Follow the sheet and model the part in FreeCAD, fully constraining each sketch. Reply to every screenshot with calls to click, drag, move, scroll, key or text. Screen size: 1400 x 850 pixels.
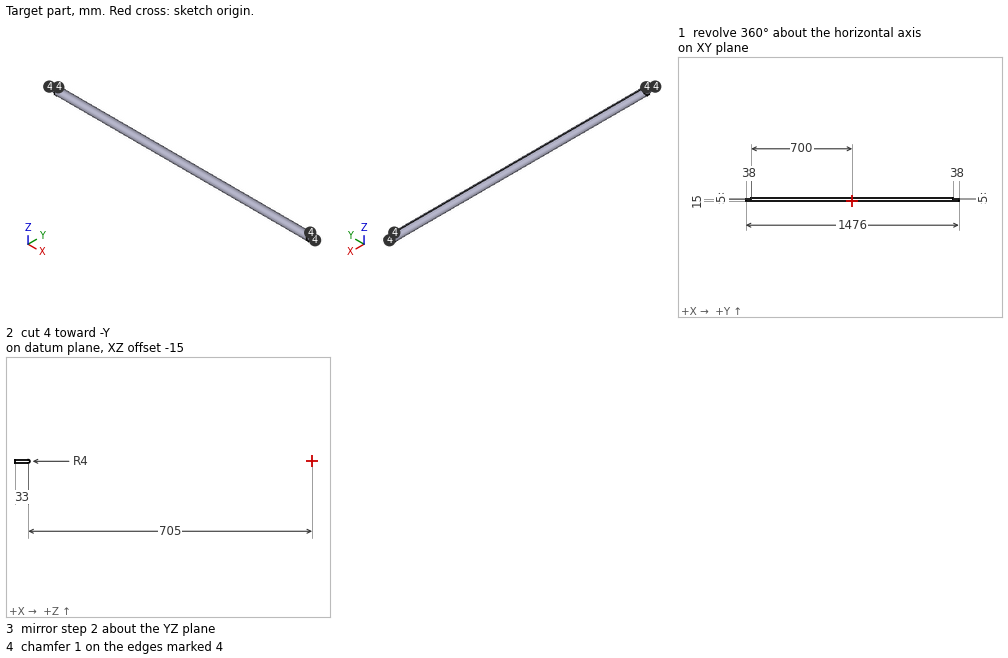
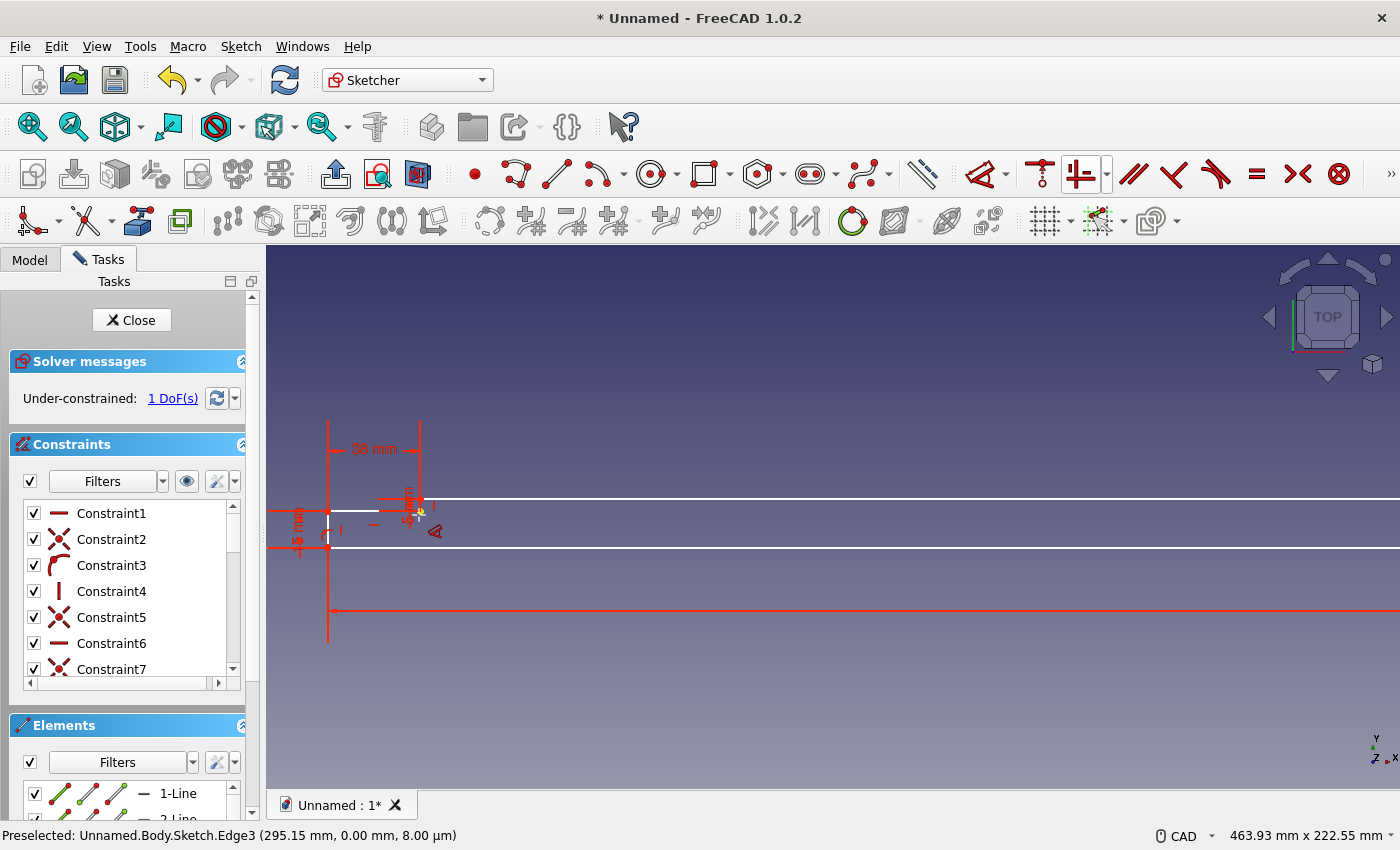
click(420, 511)
click(828, 582)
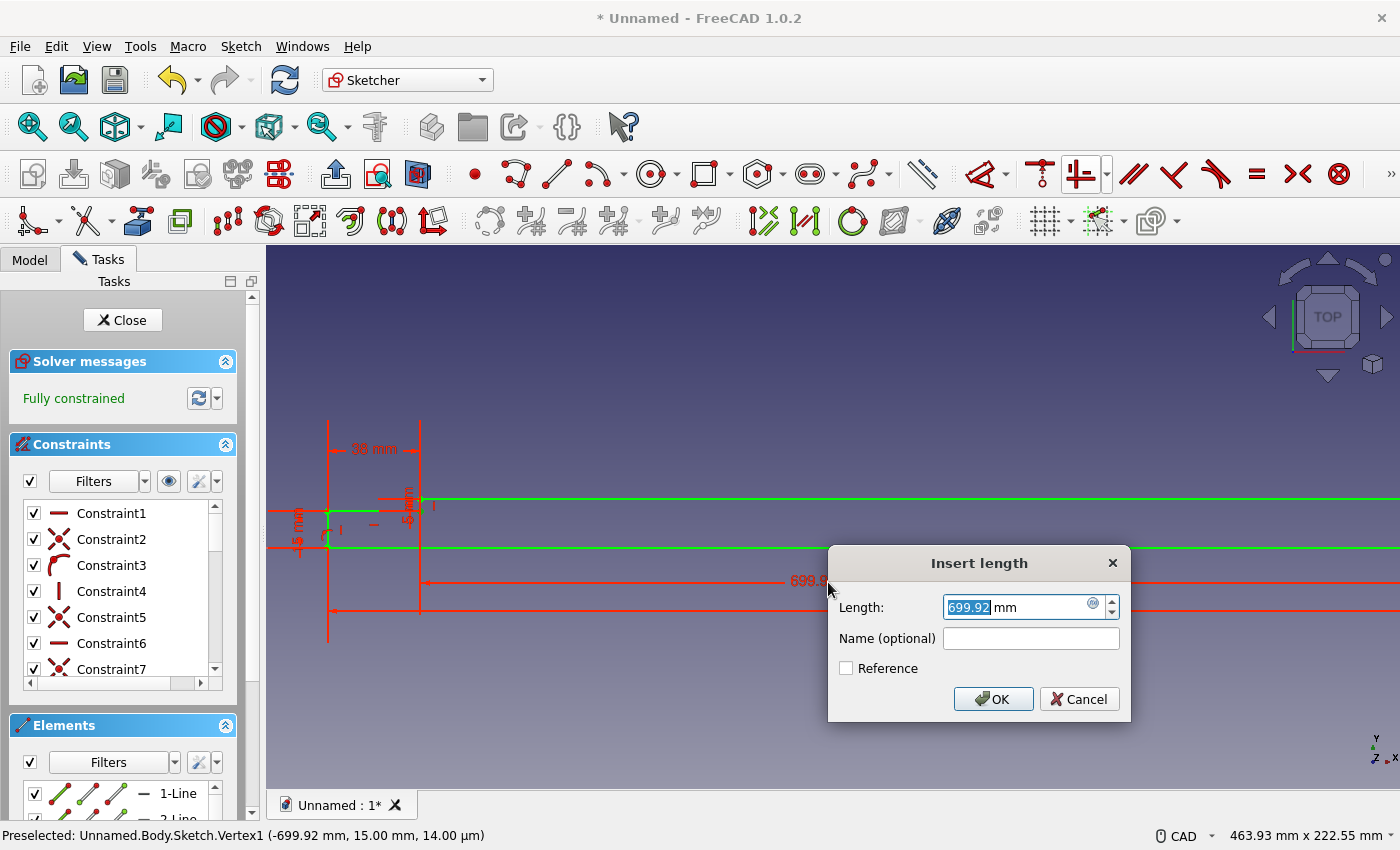
text(700)
key(Return)
key(Escape)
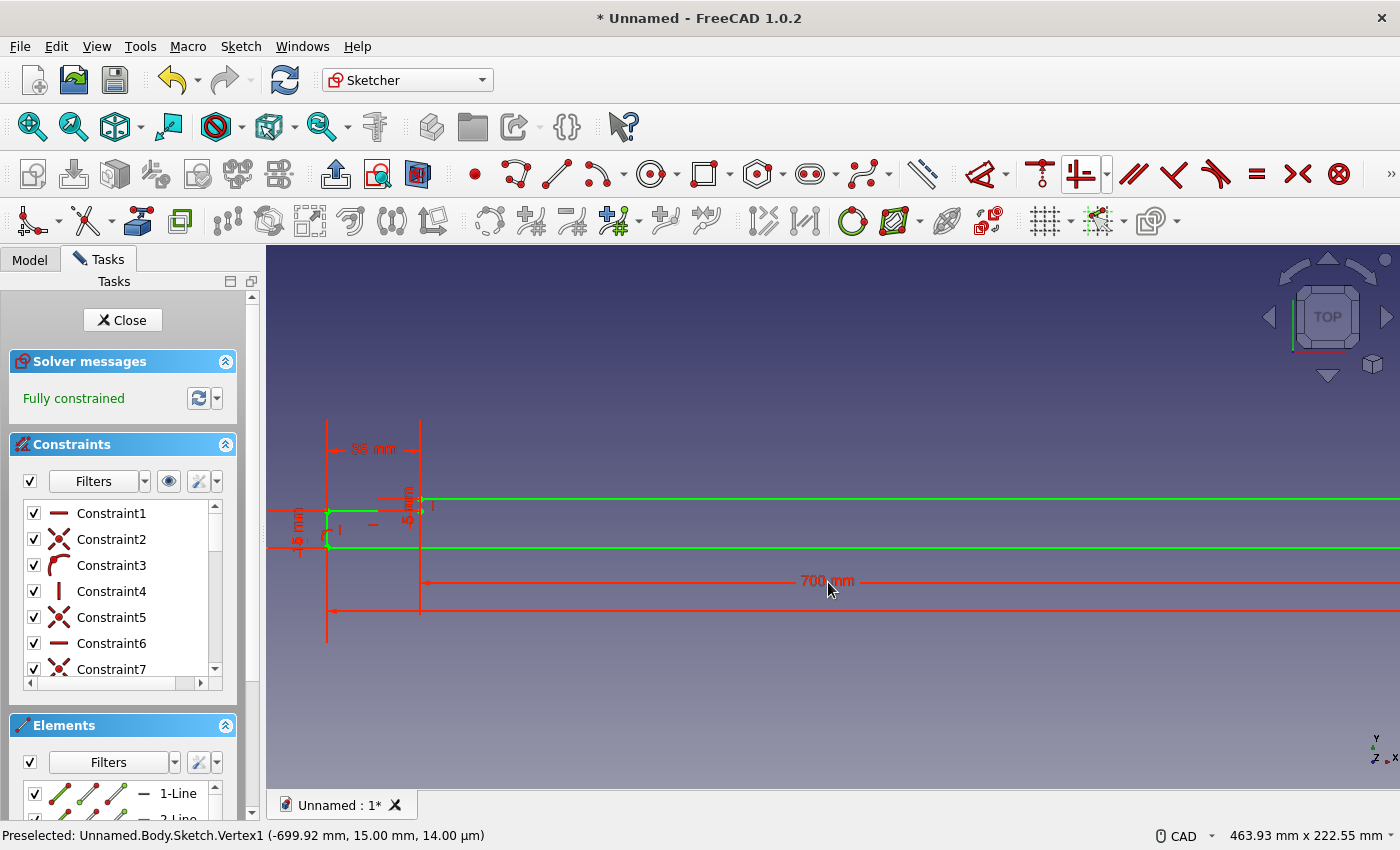
click(123, 320)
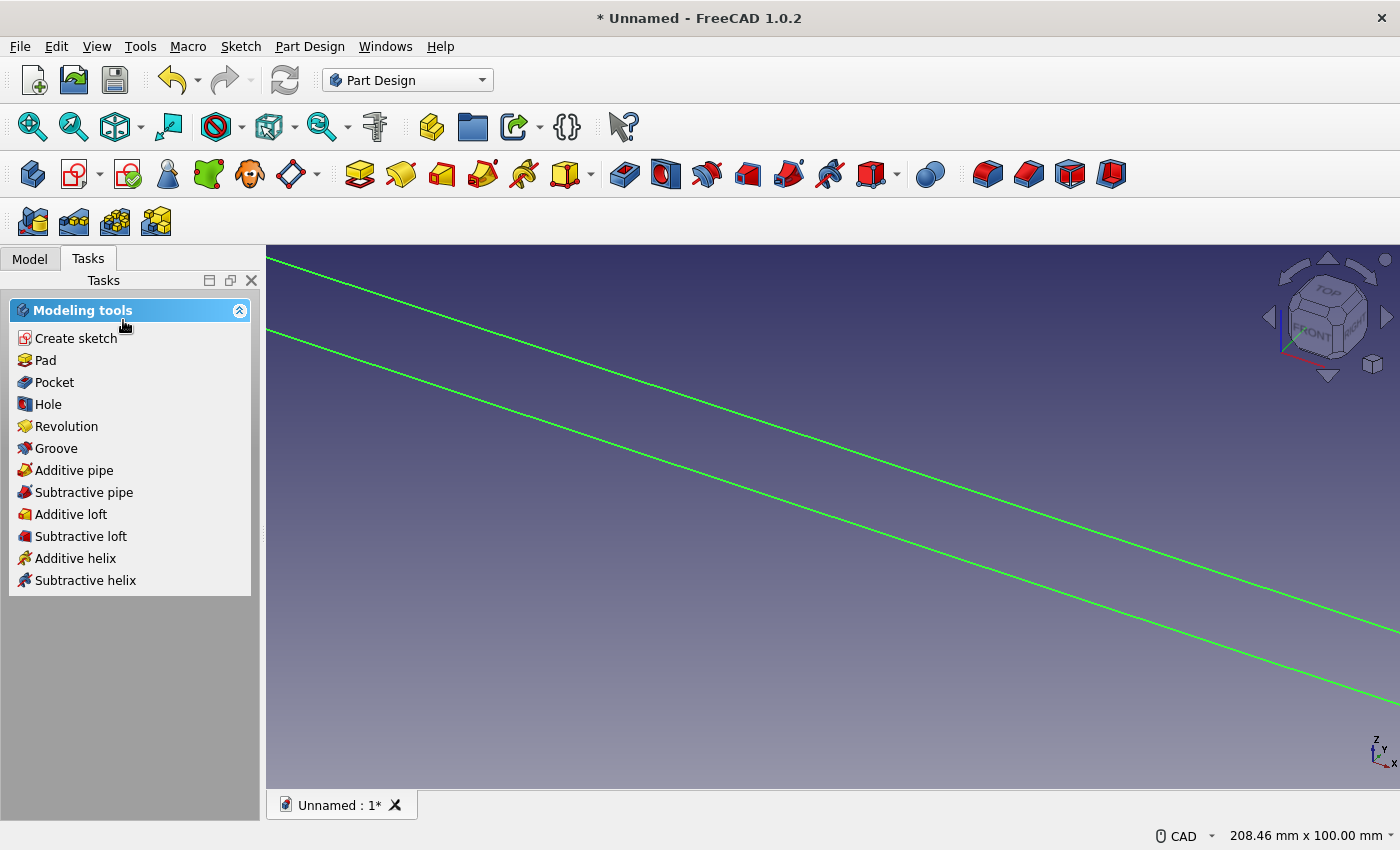
click(401, 174)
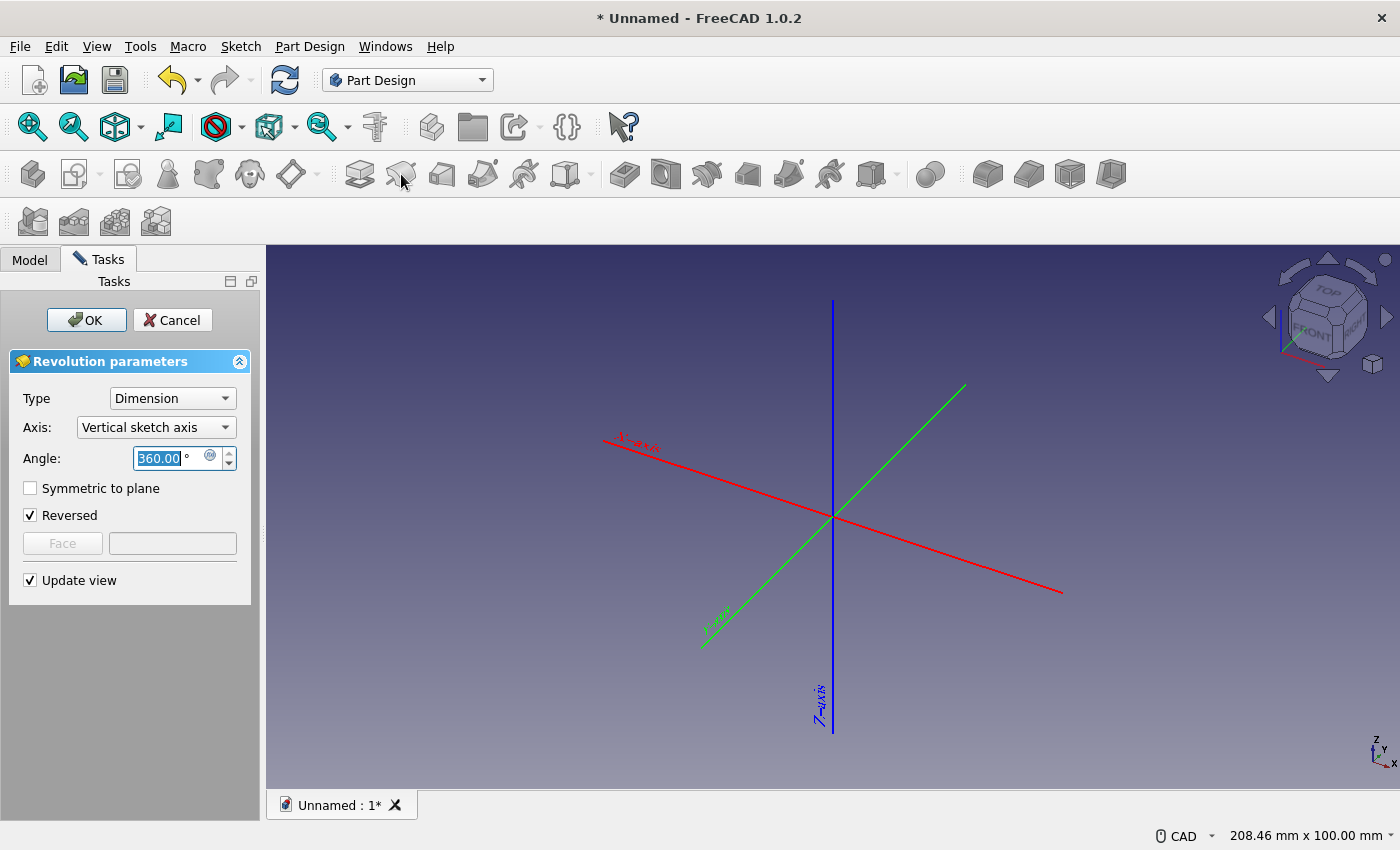
click(157, 428)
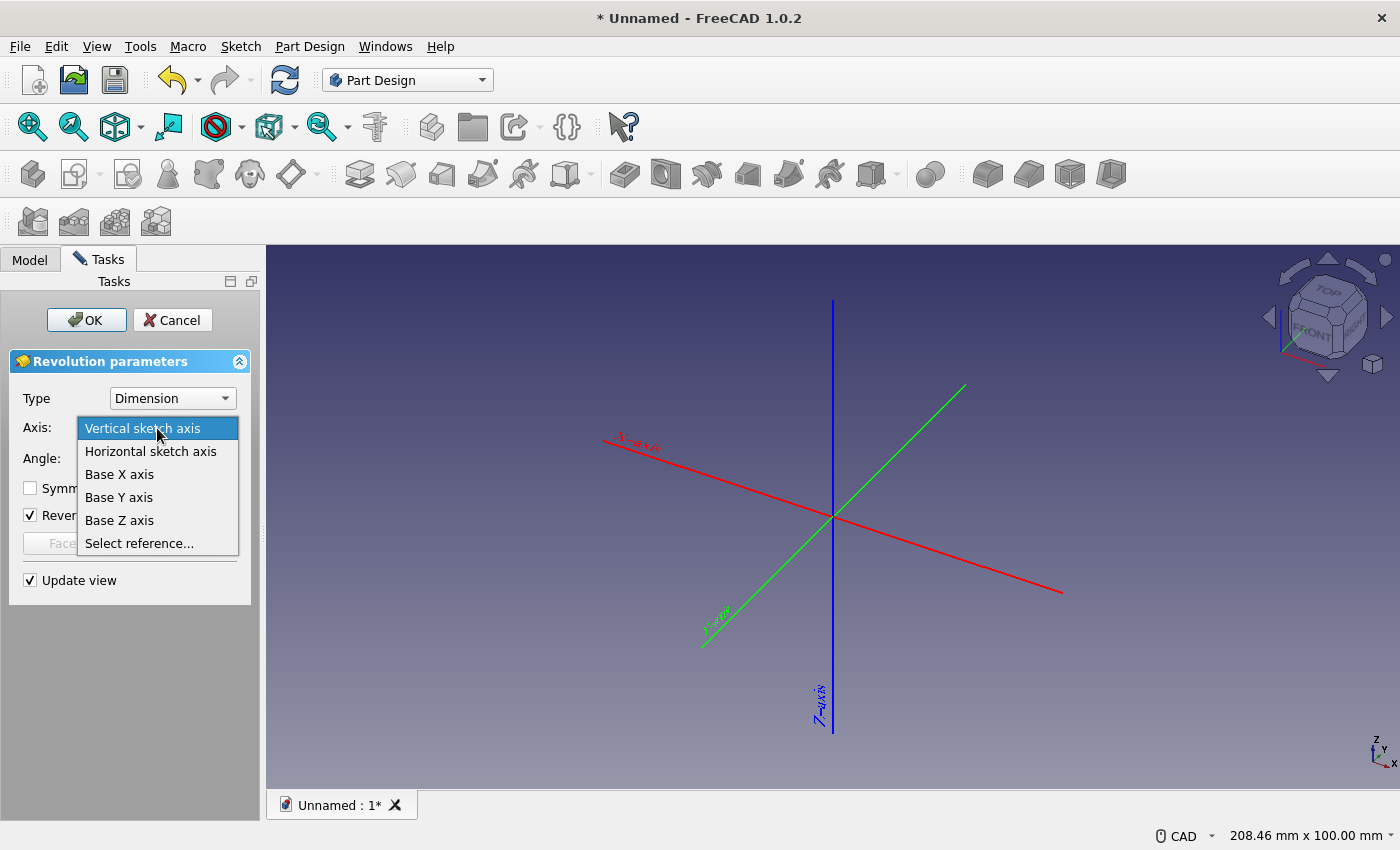
click(156, 452)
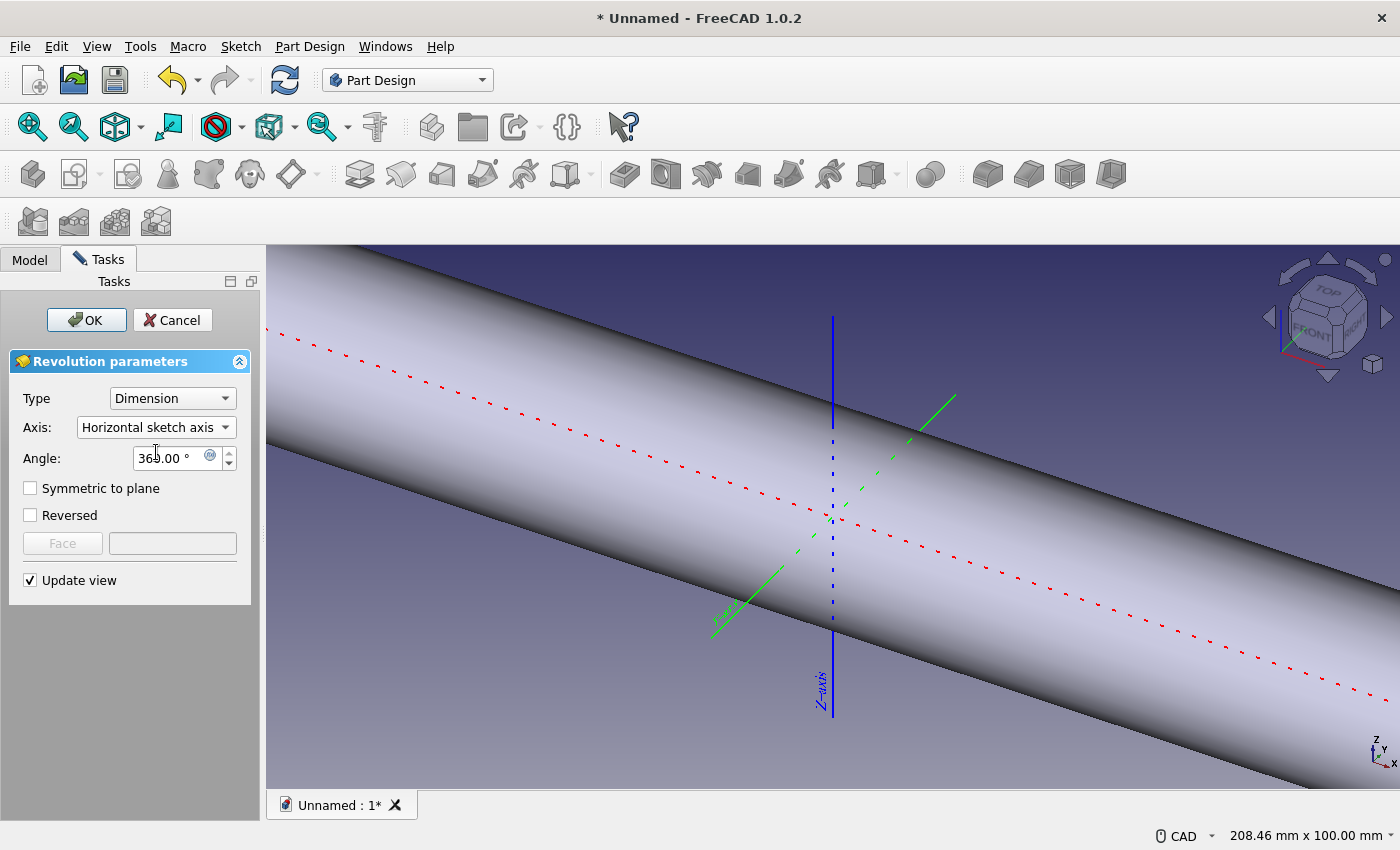
click(87, 320)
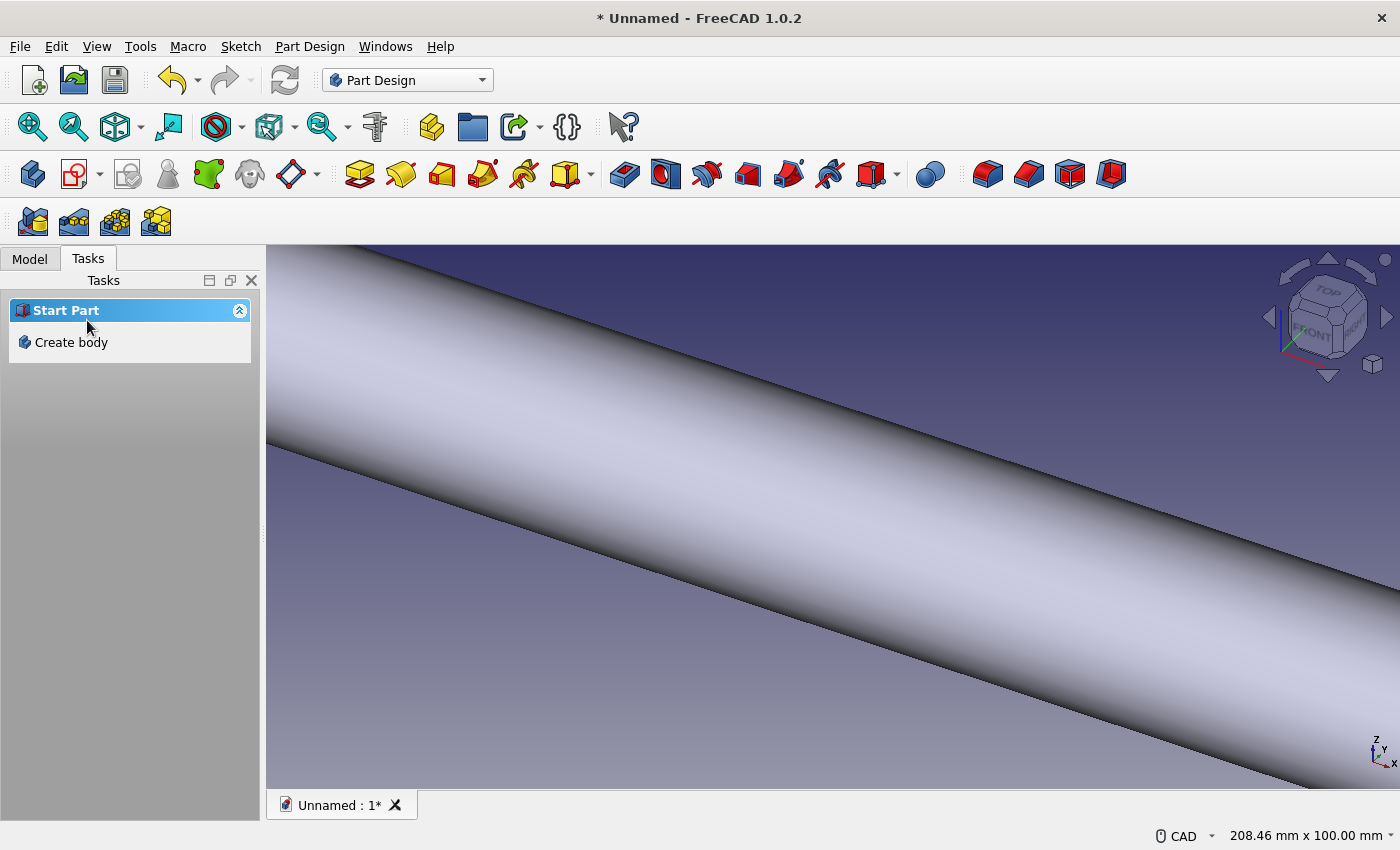
click(33, 128)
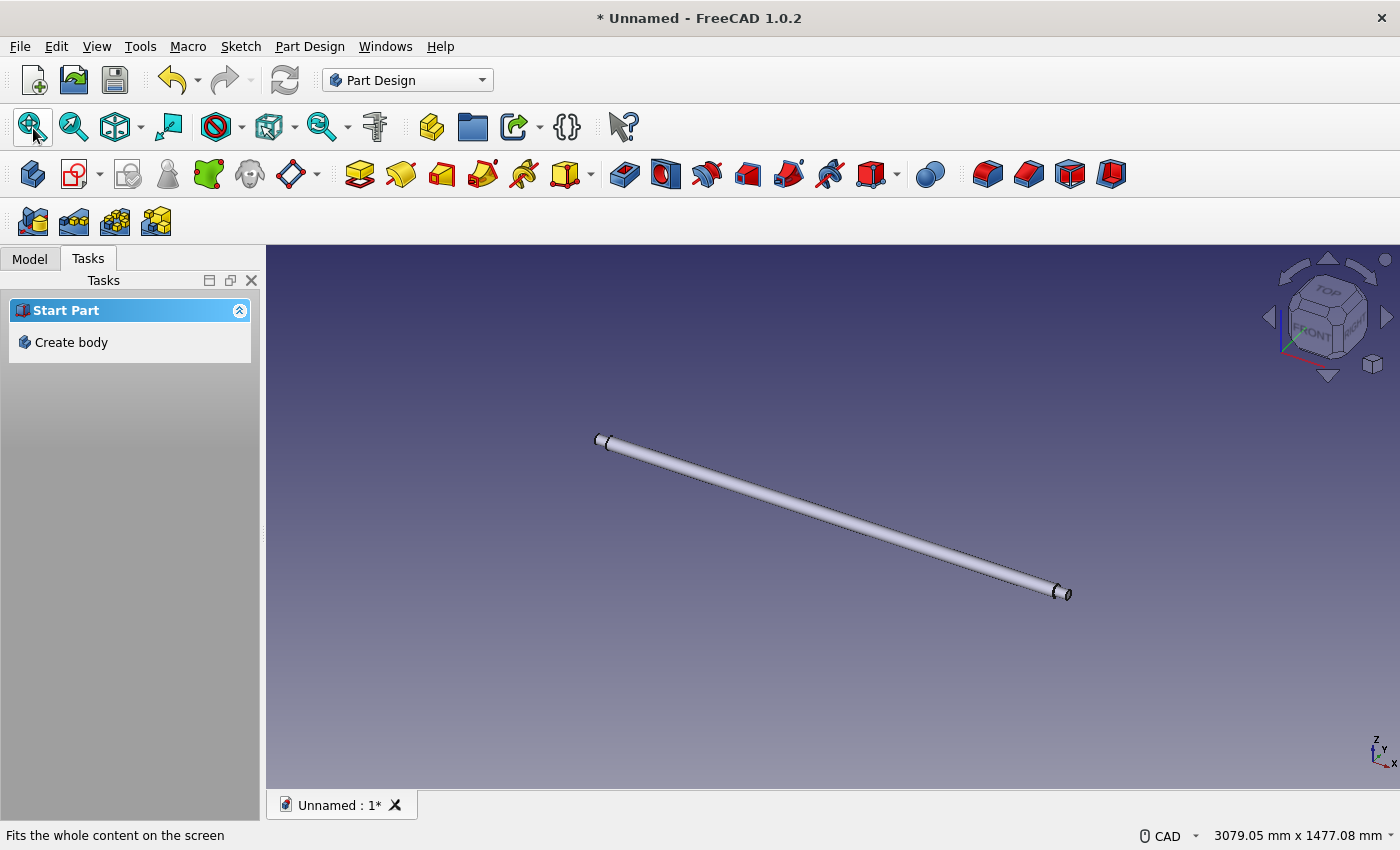
click(30, 258)